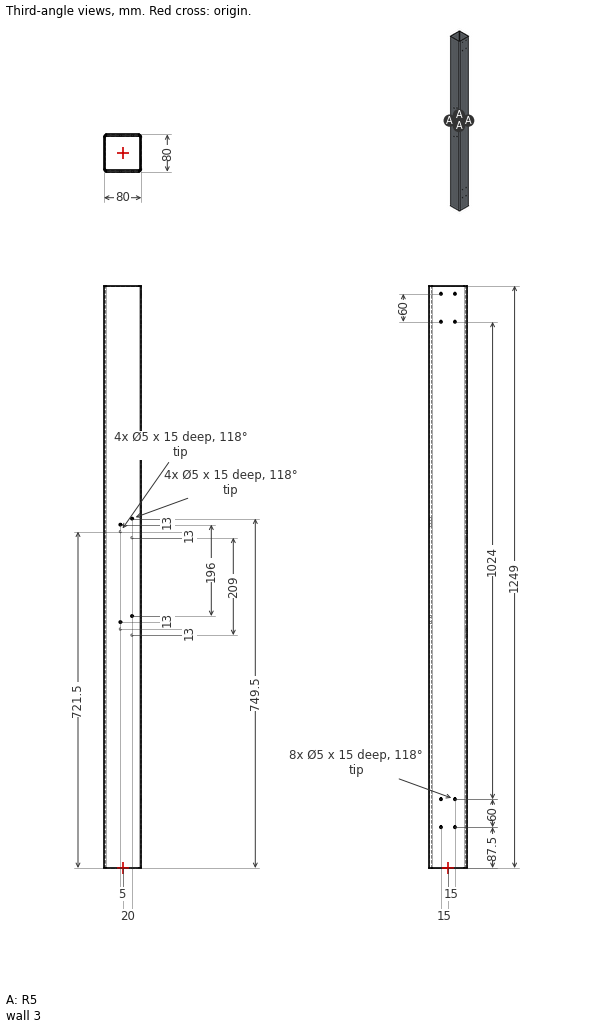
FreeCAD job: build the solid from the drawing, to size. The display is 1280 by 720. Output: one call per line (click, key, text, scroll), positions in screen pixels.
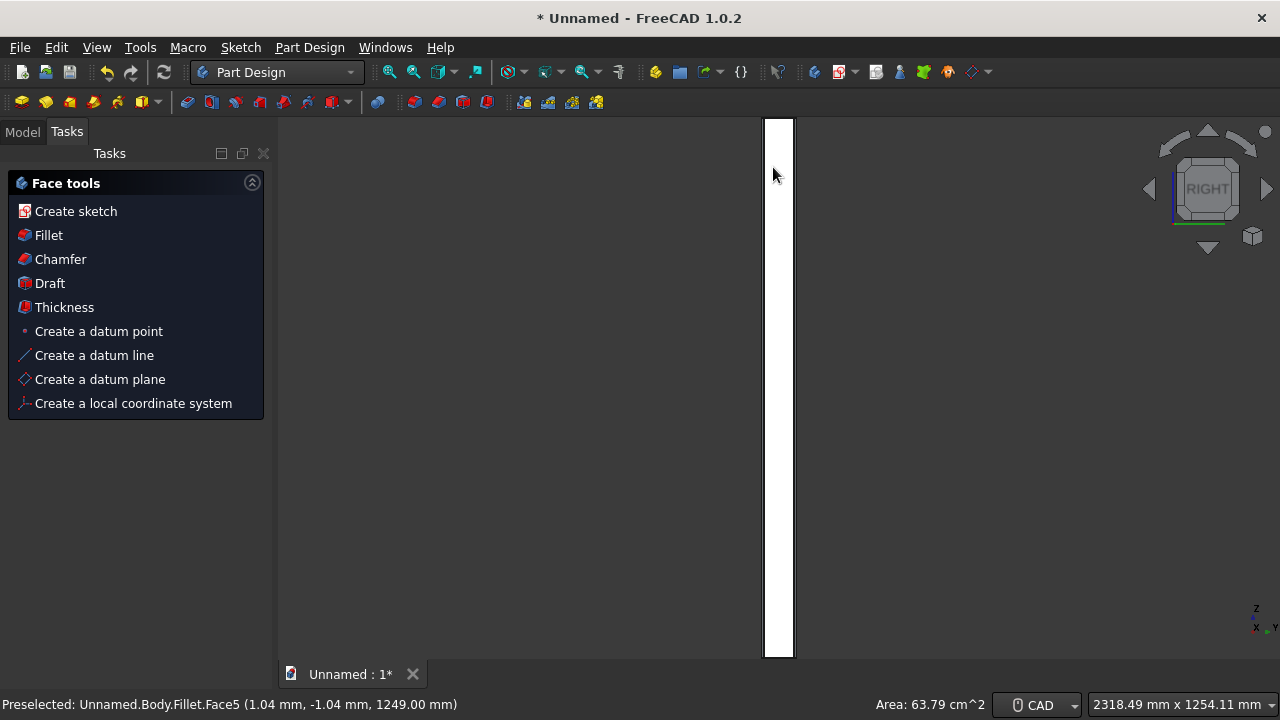
key(5)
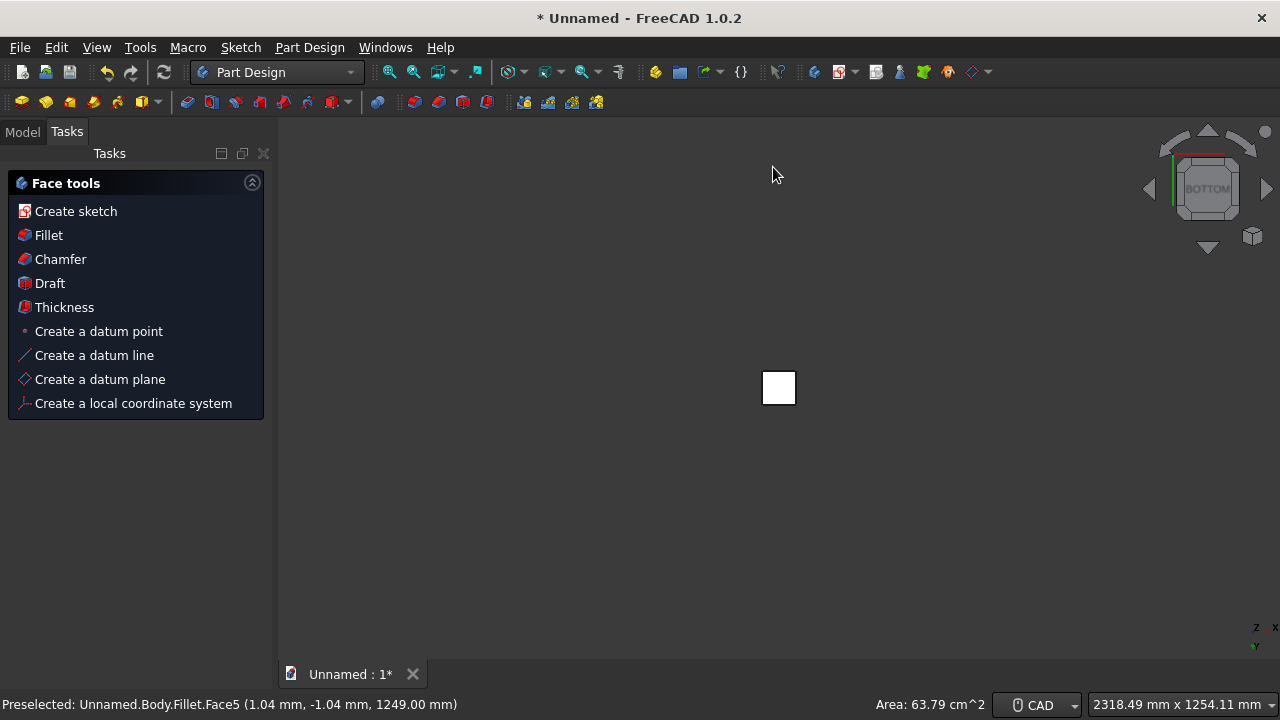
click(390, 72)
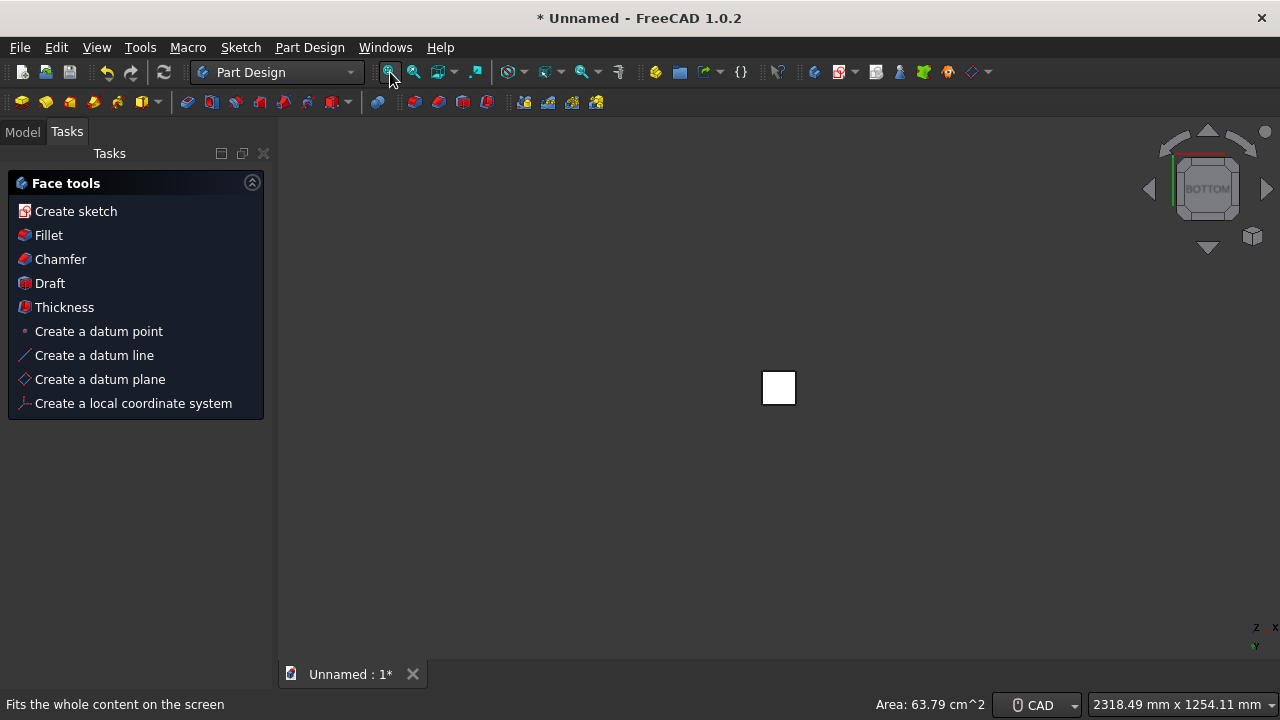
click(779, 387, ctrl)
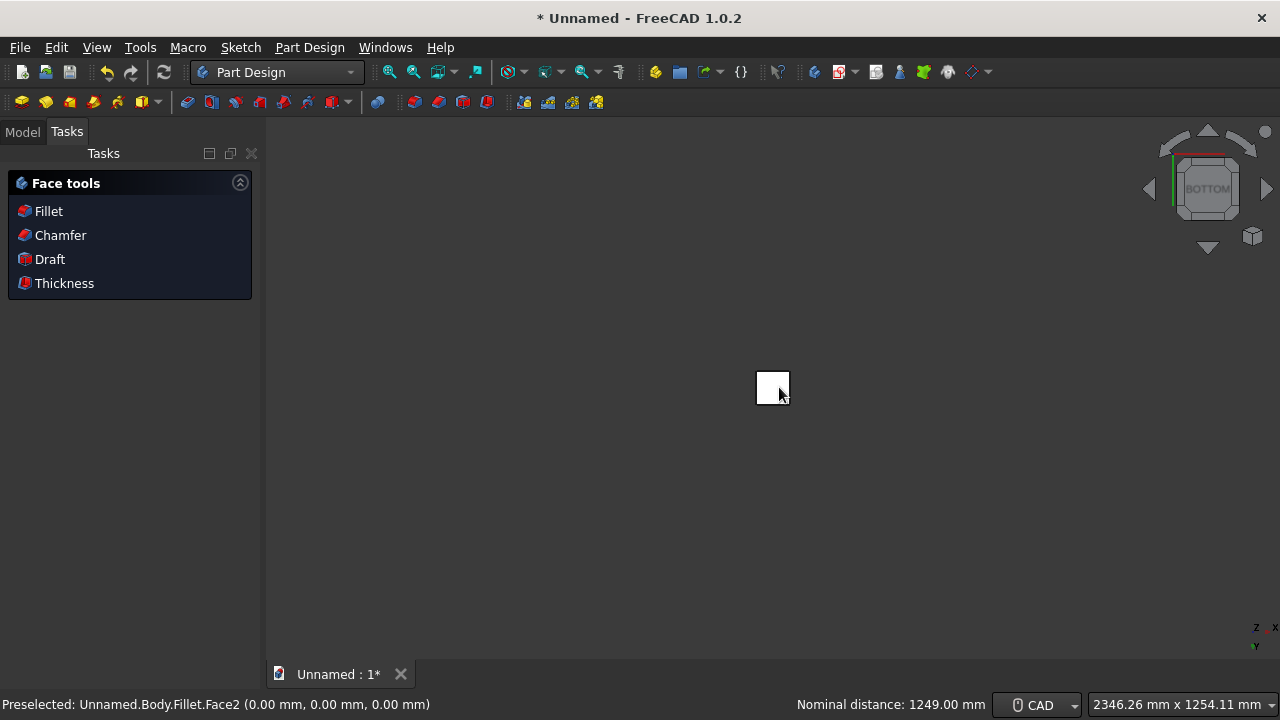
click(488, 102)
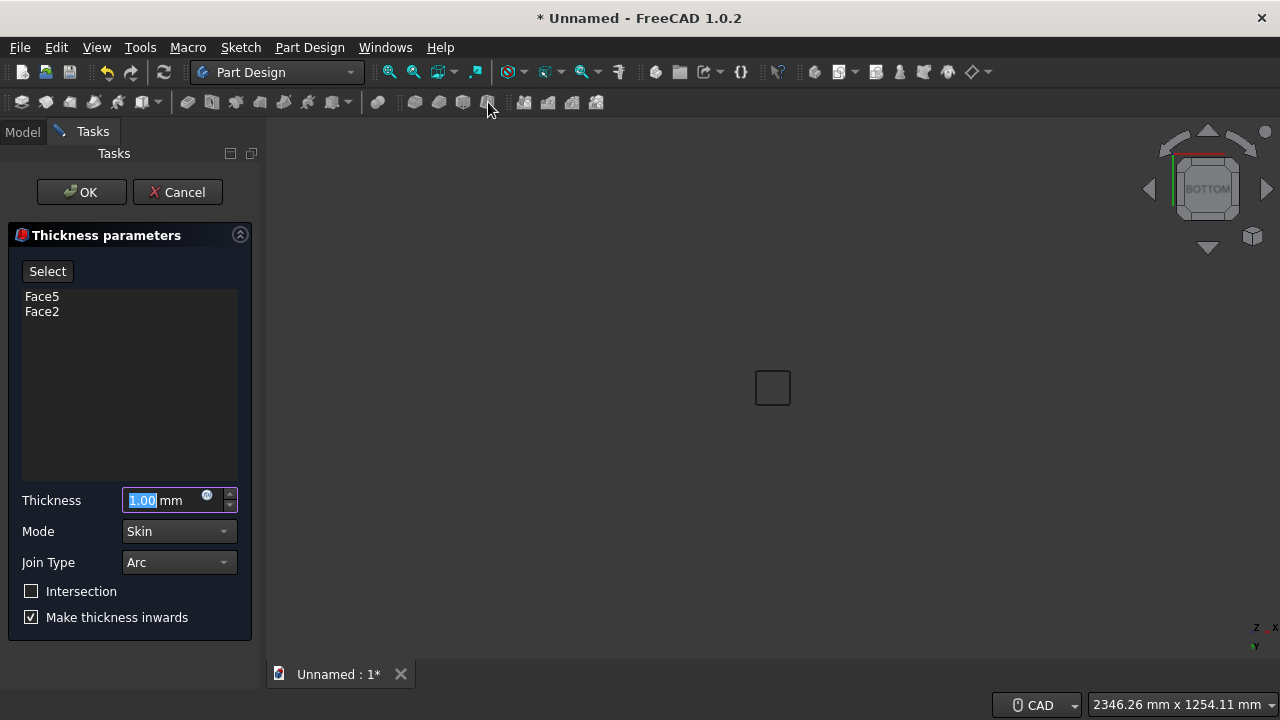
text(3)
key(Tab)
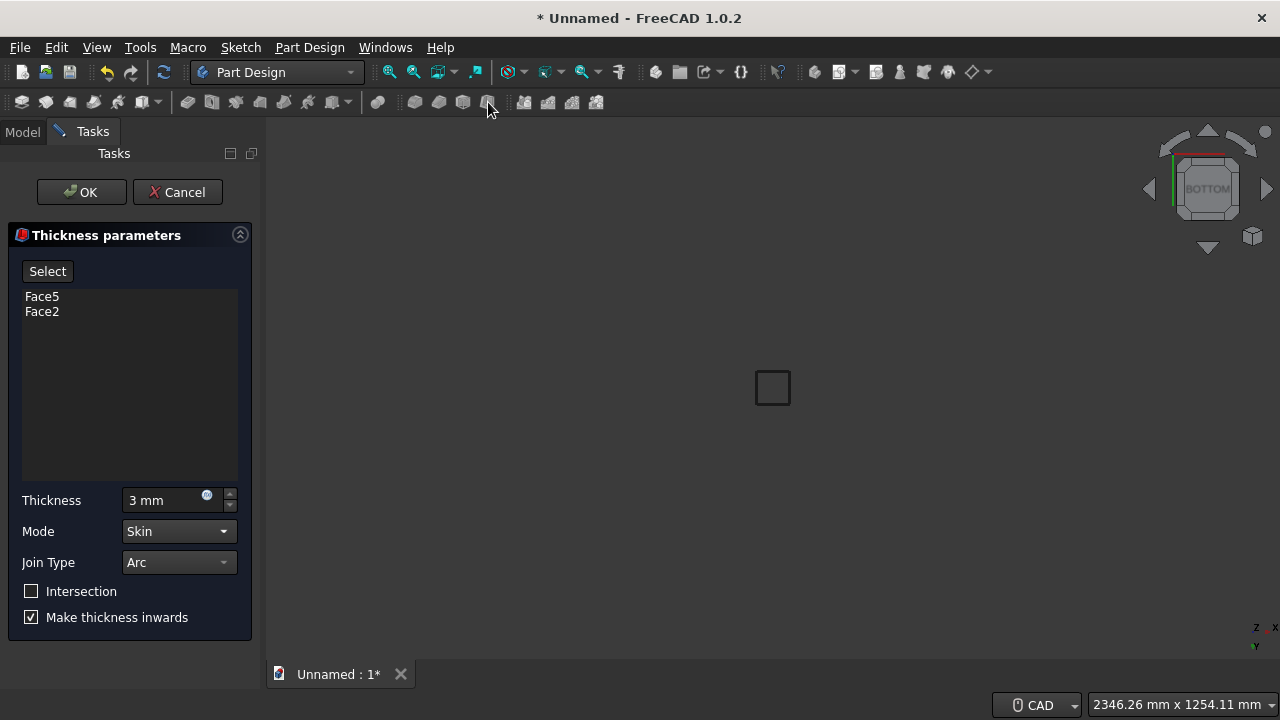
click(180, 562)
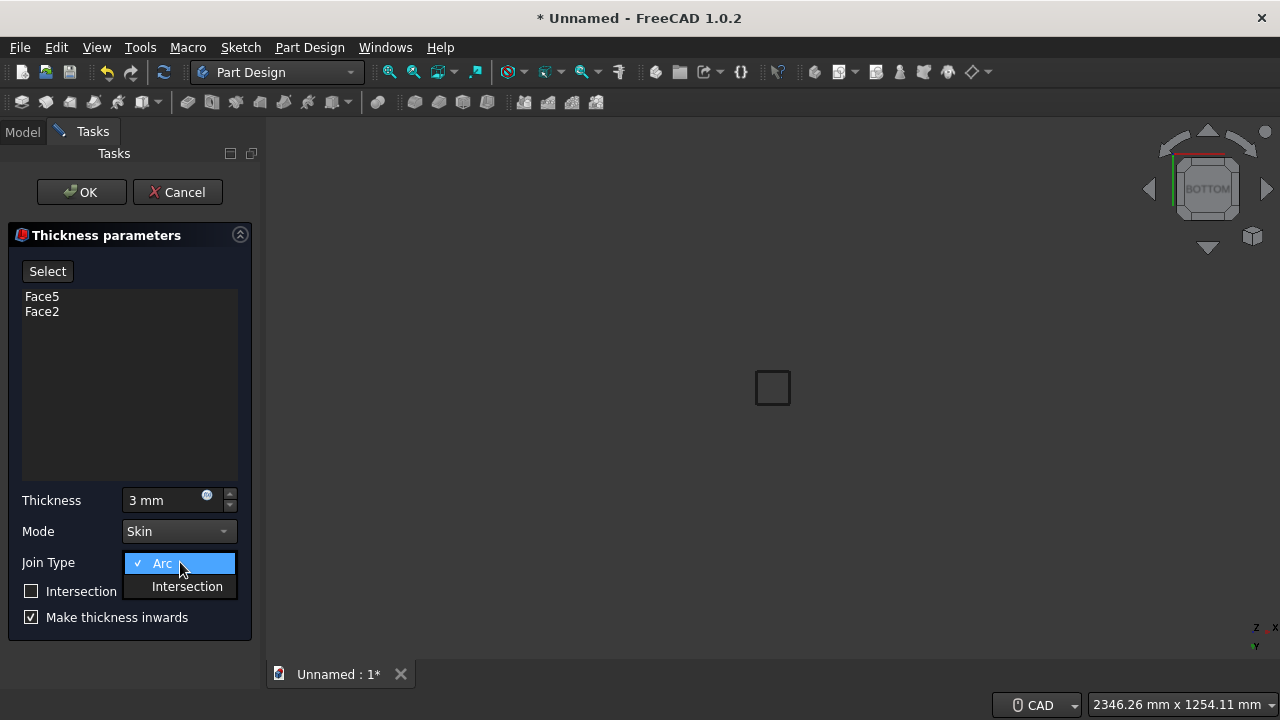
click(179, 586)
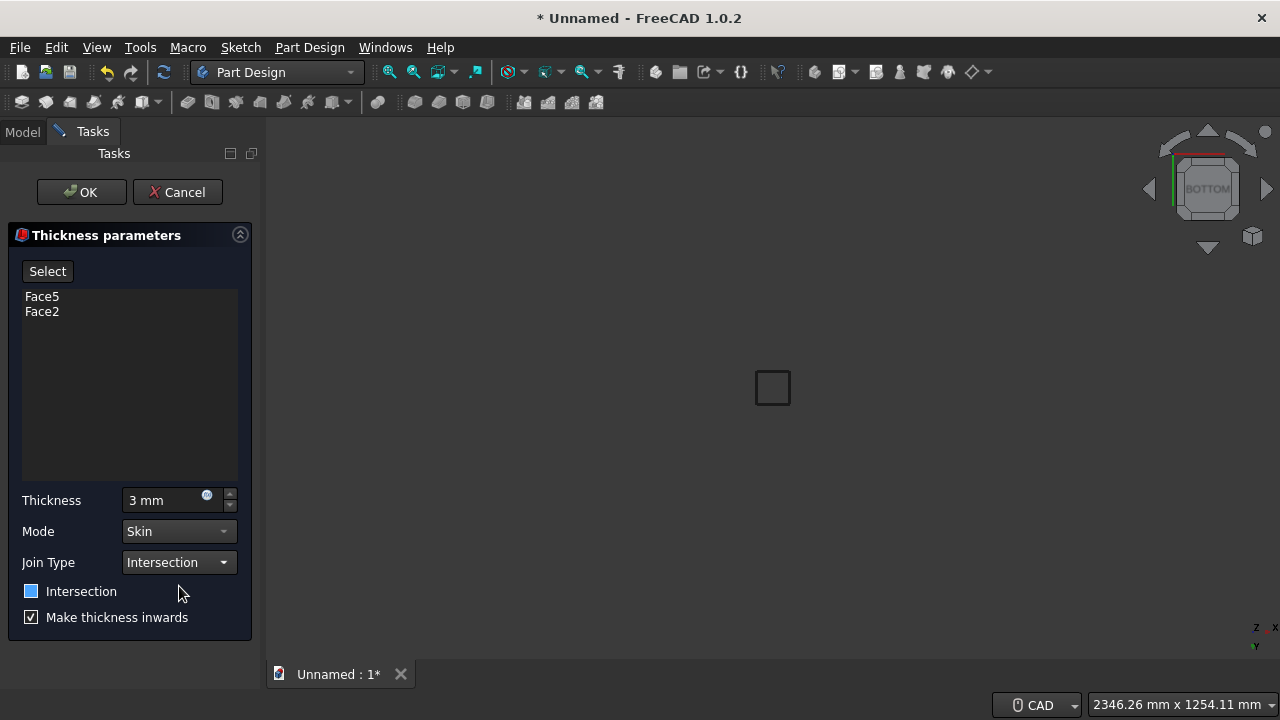
click(82, 192)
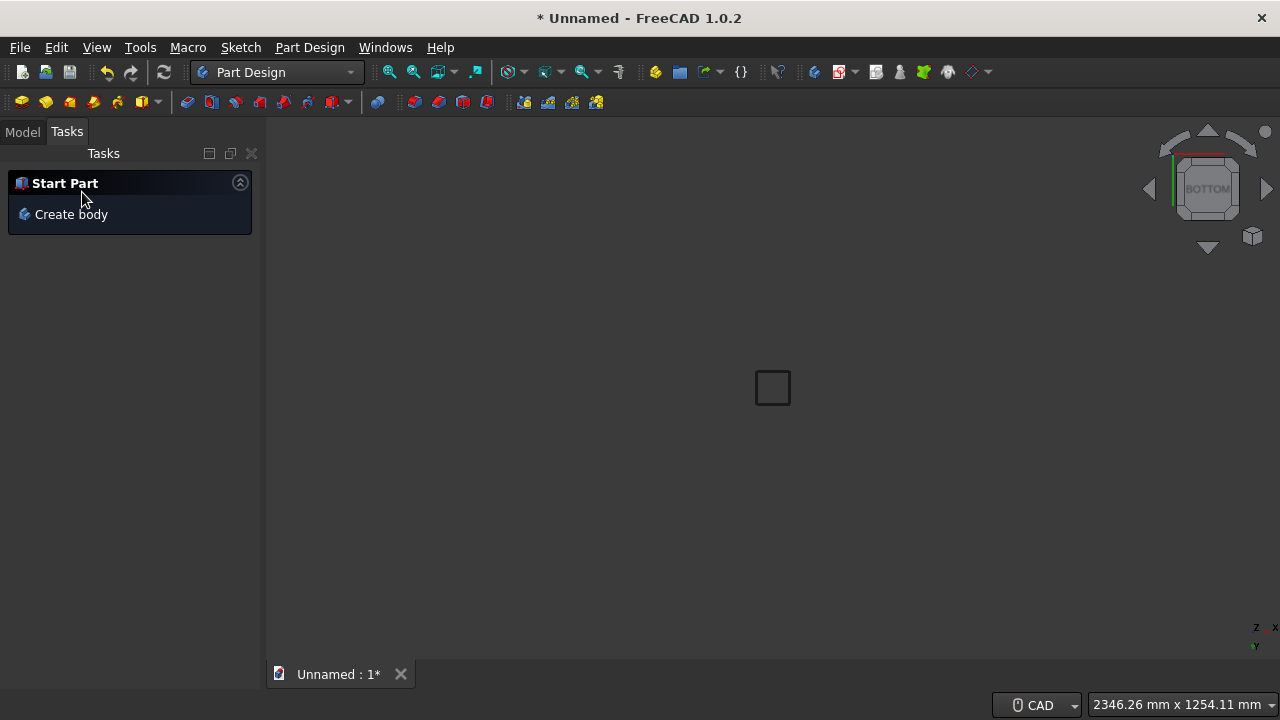
key(v)
key(f)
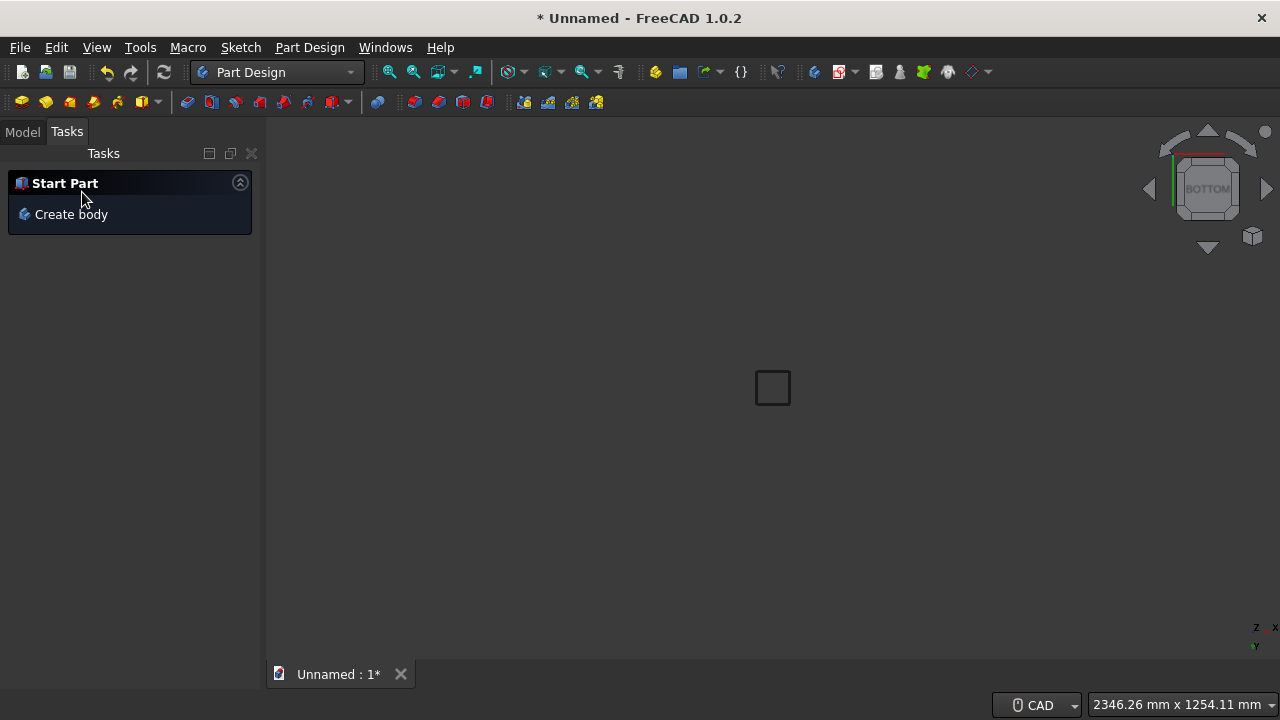
key(0)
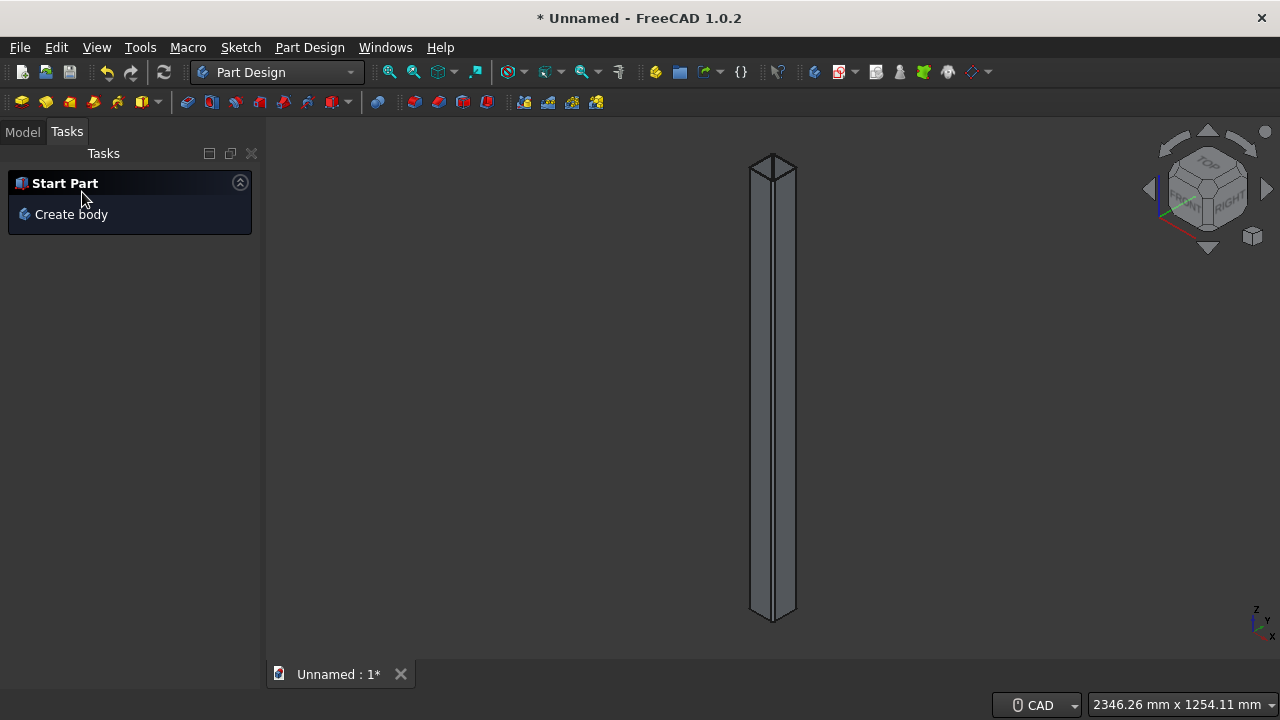
click(785, 205)